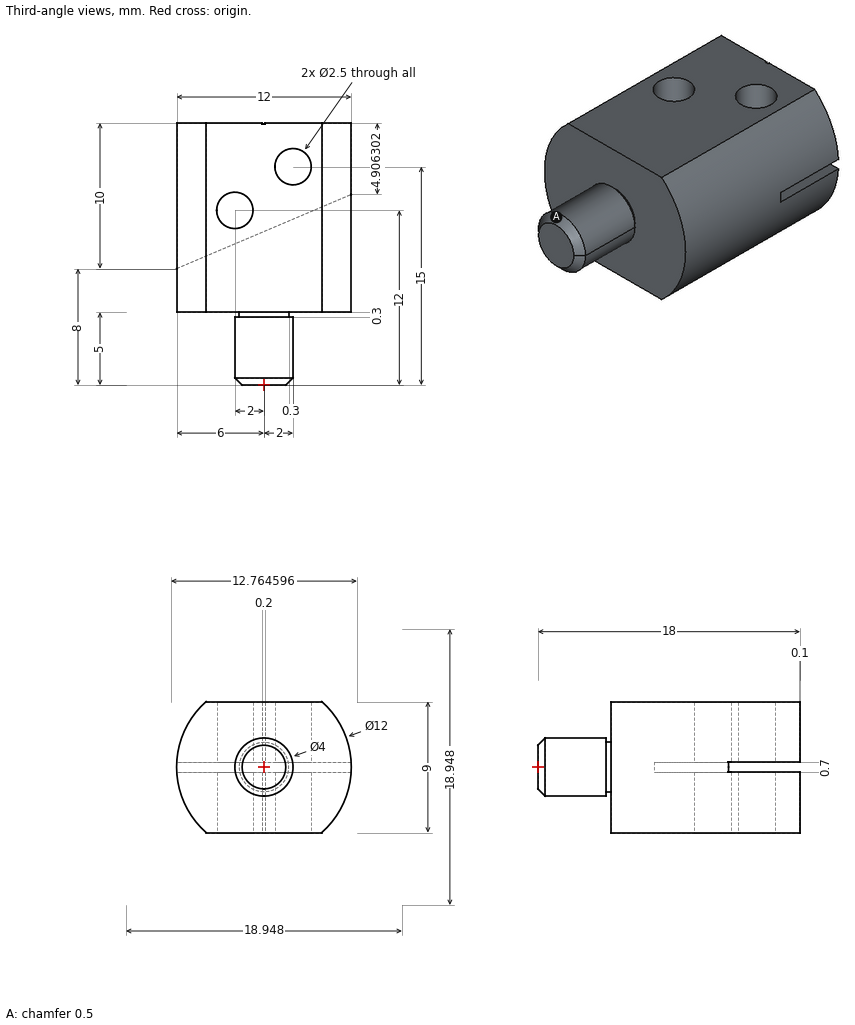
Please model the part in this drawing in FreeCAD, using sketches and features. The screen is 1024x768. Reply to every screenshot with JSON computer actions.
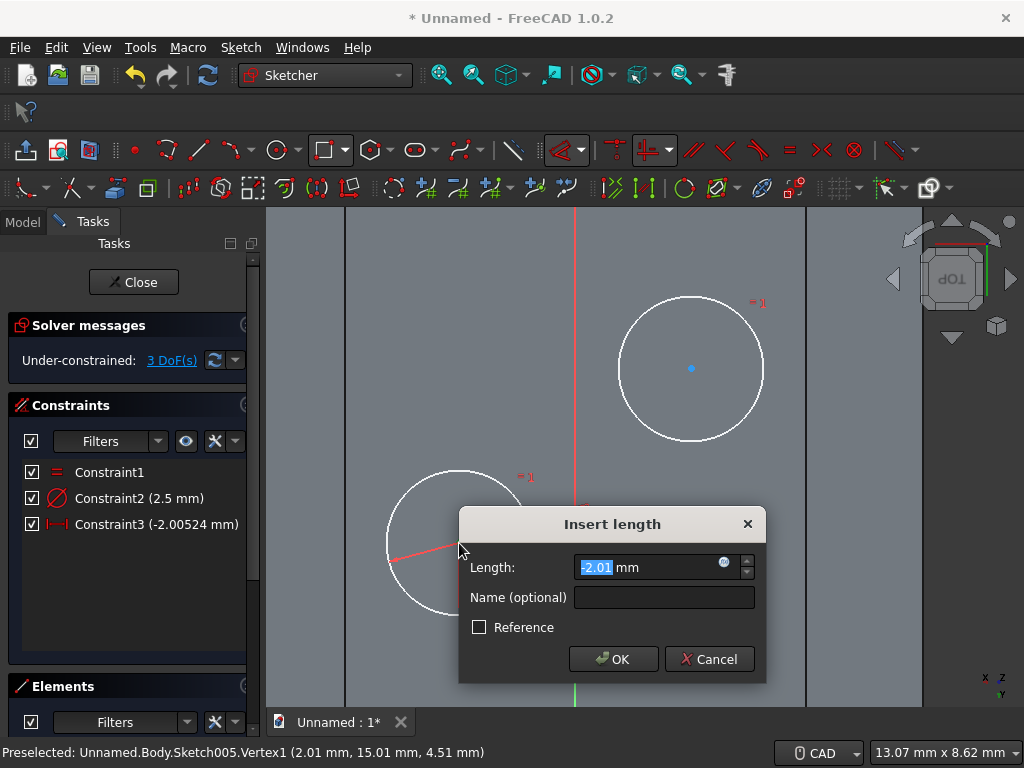
{"action": "type", "text": "-2"}
{"action": "key", "text": "Return"}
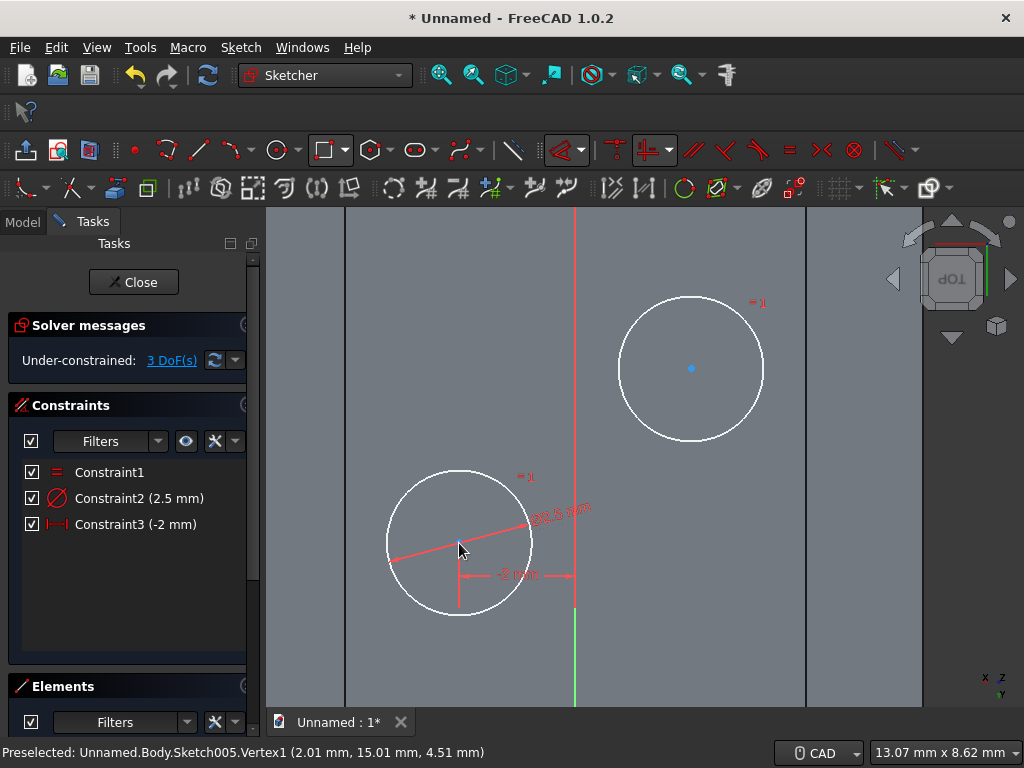
{"action": "left_click", "coordinate": [691, 369]}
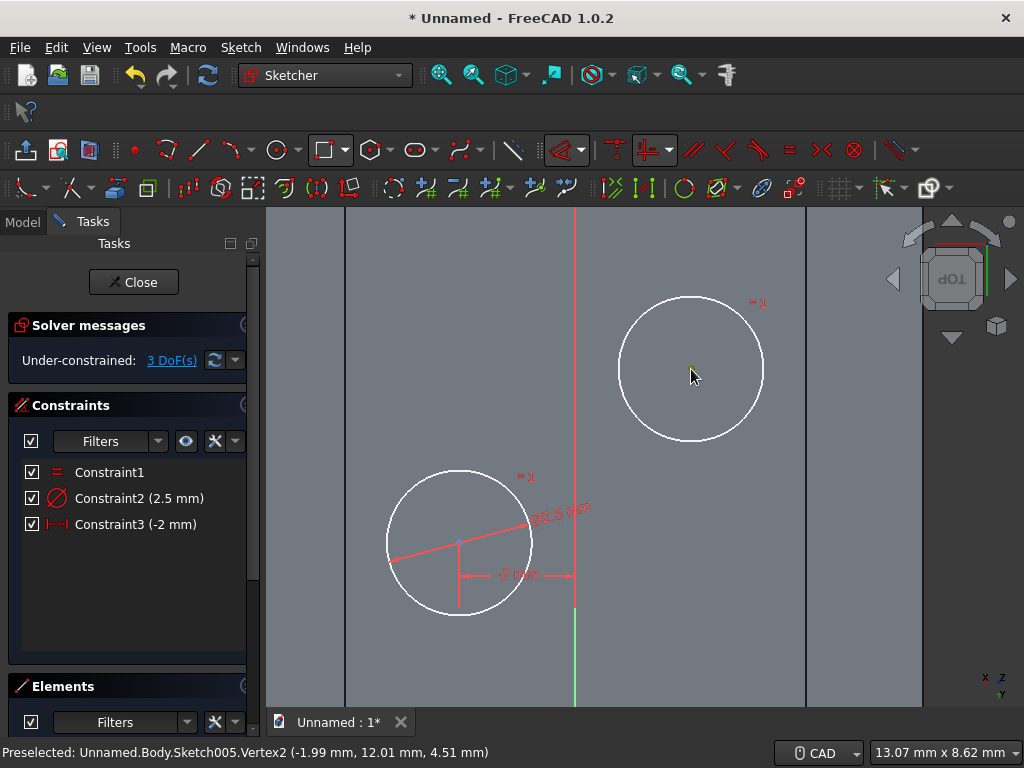
{"action": "key", "text": "l"}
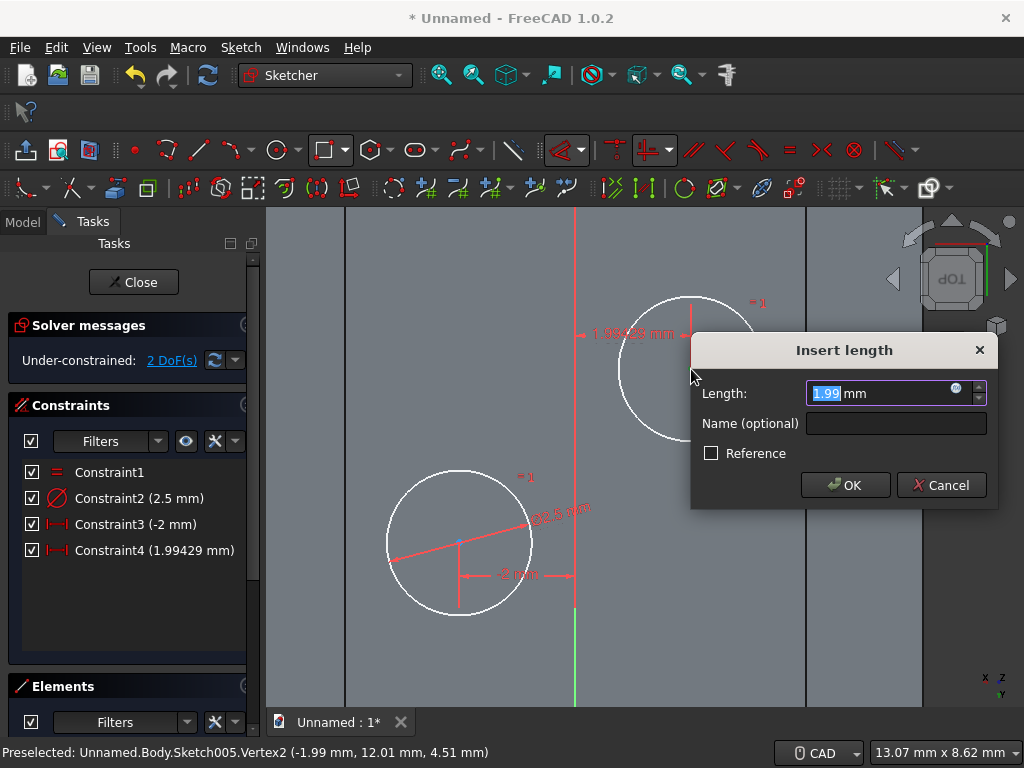
{"action": "type", "text": "2"}
{"action": "key", "text": "Return"}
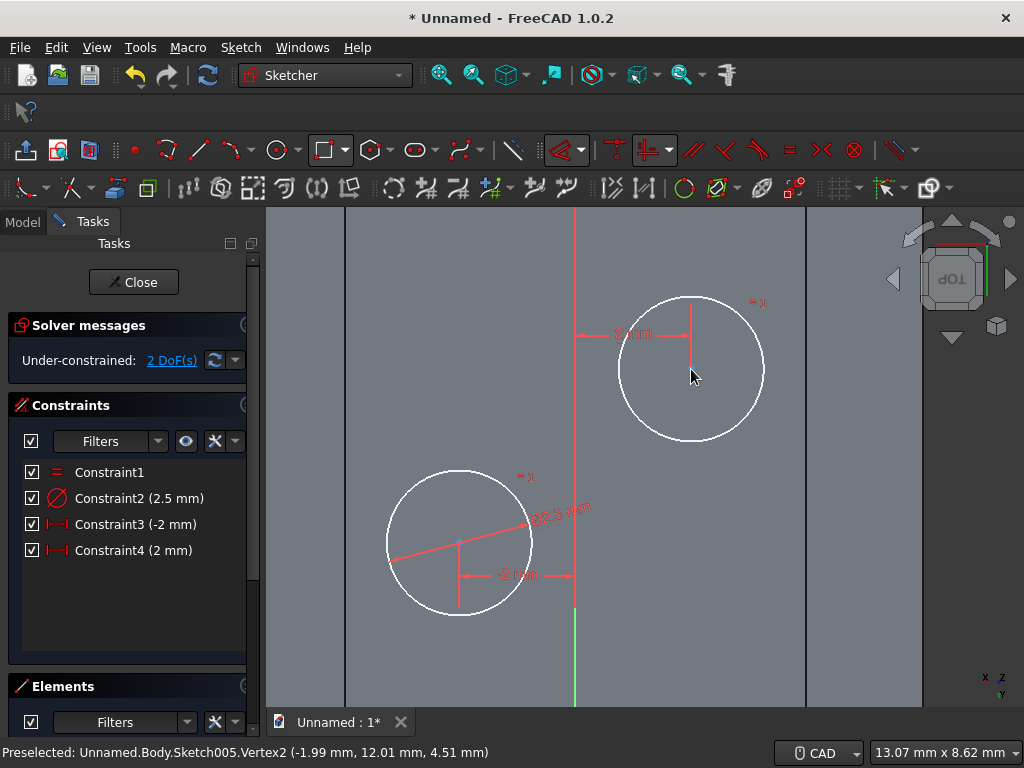
{"action": "left_click", "coordinate": [459, 543]}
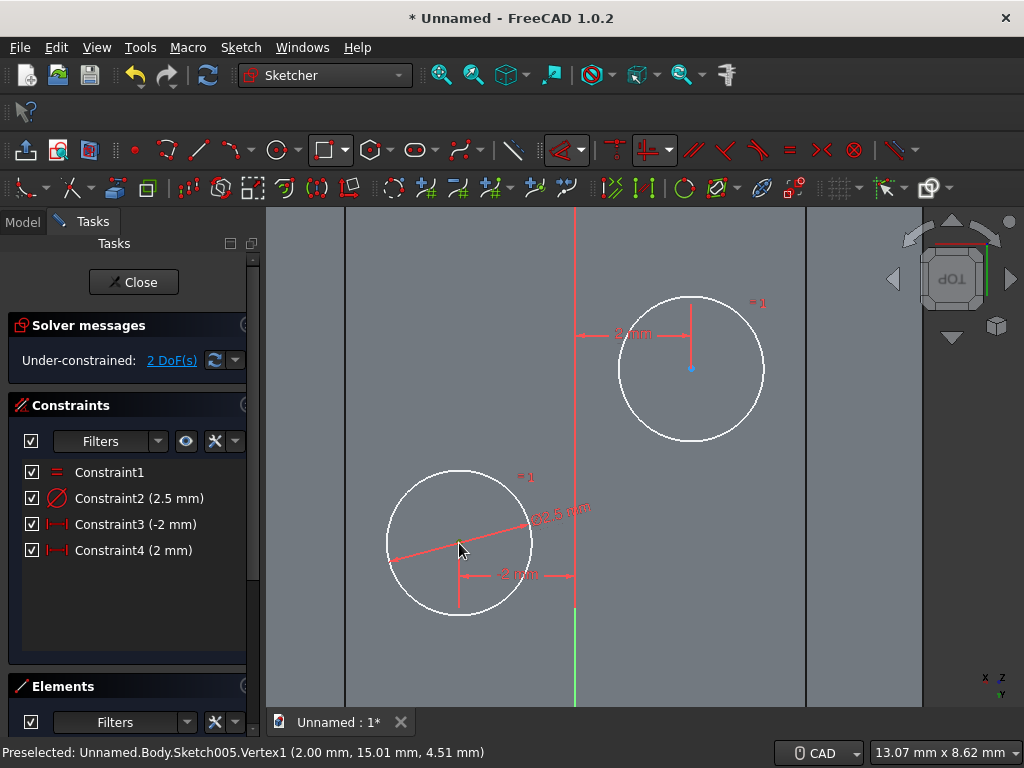
{"action": "key", "text": "i"}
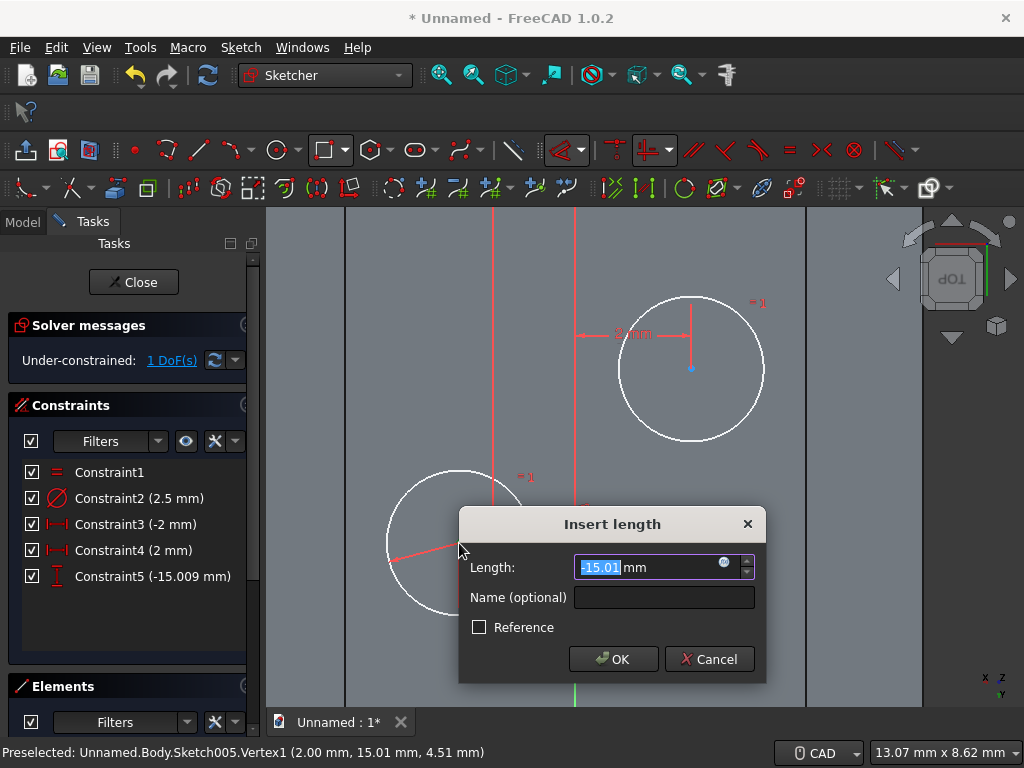
{"action": "type", "text": "-15"}
{"action": "key", "text": "Return"}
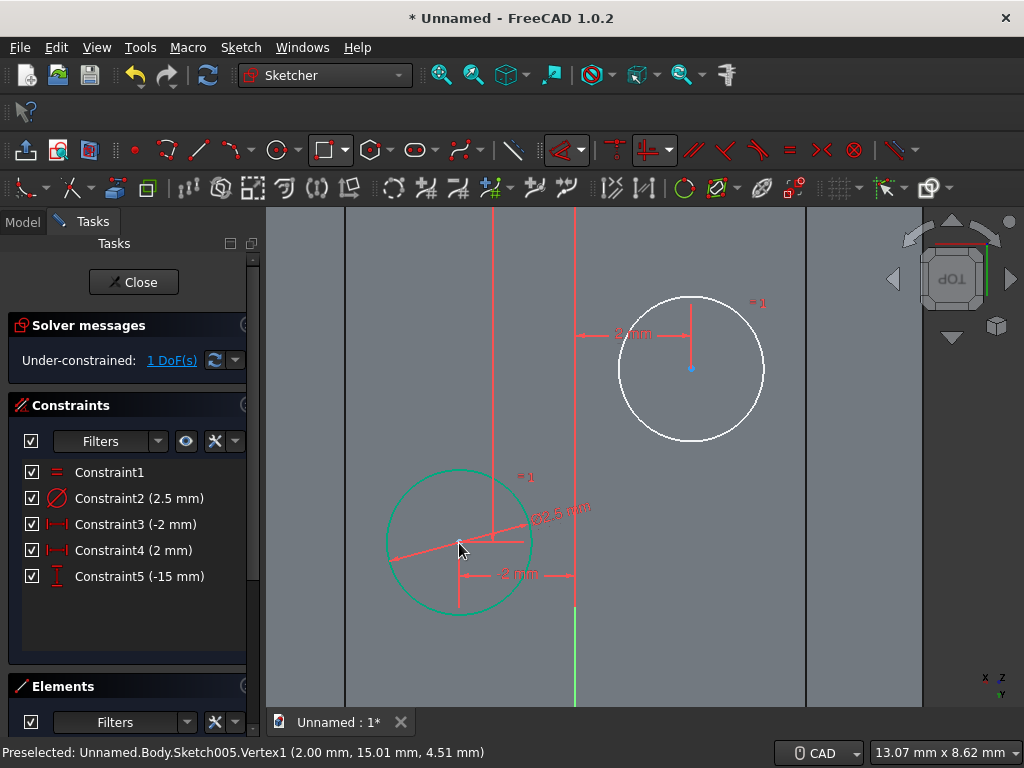
{"action": "left_click", "coordinate": [691, 369]}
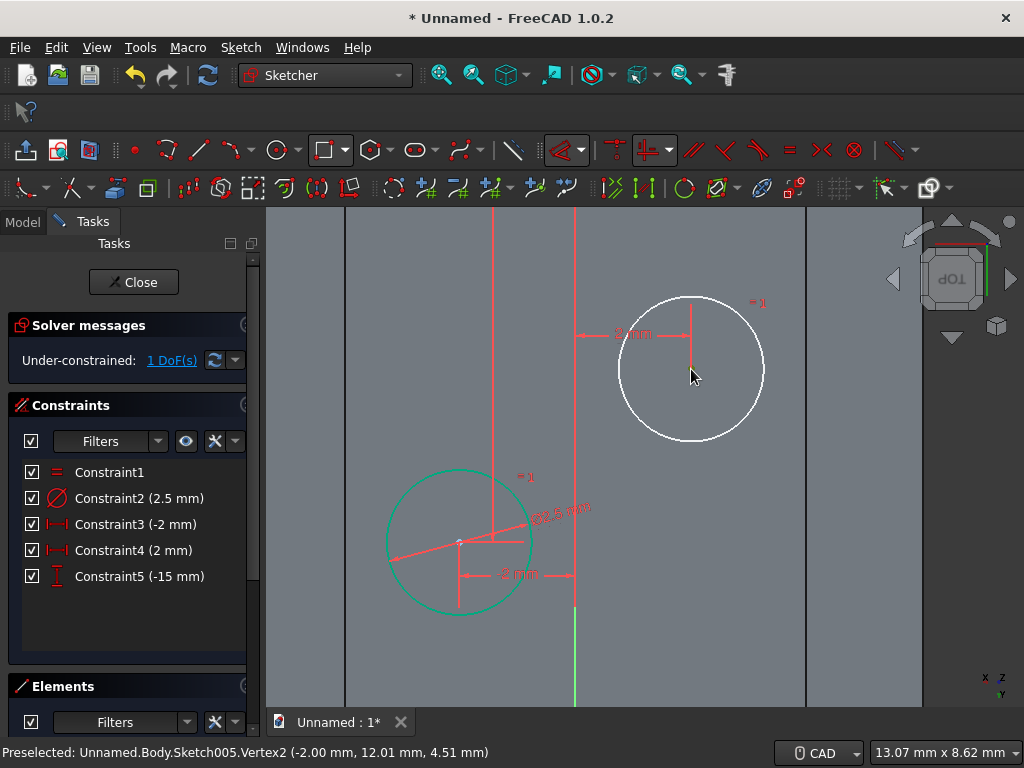
{"action": "key", "text": "i"}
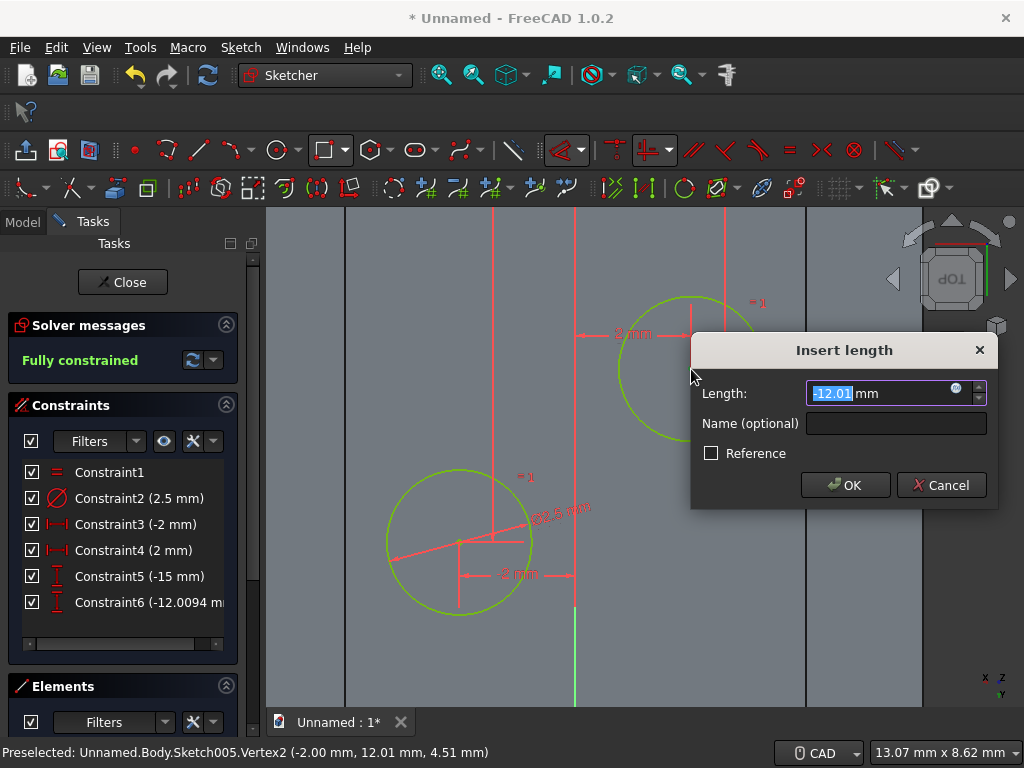
{"action": "type", "text": "-12"}
{"action": "key", "text": "Return"}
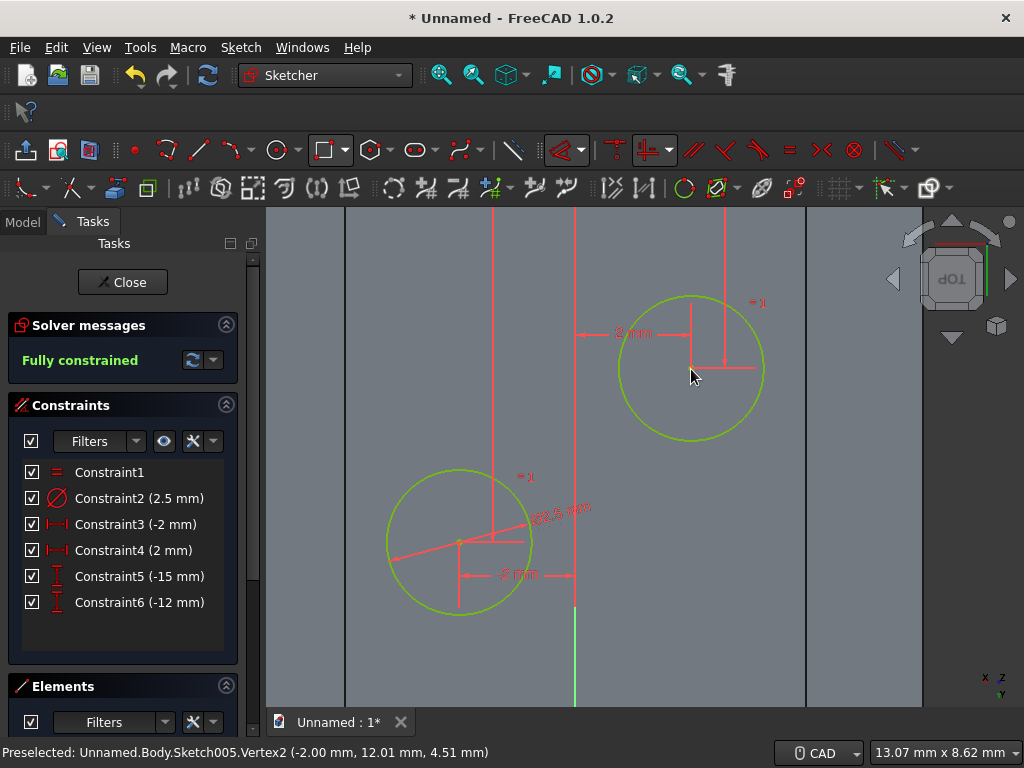
{"action": "left_click", "coordinate": [123, 282]}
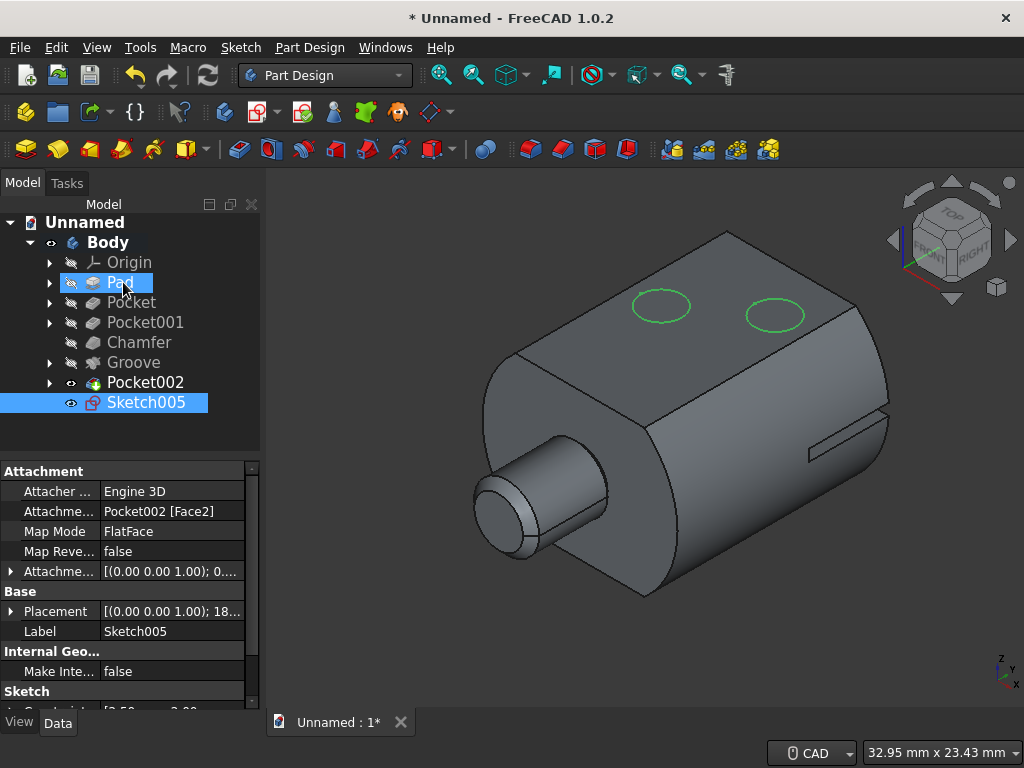
{"action": "left_click", "coordinate": [272, 150]}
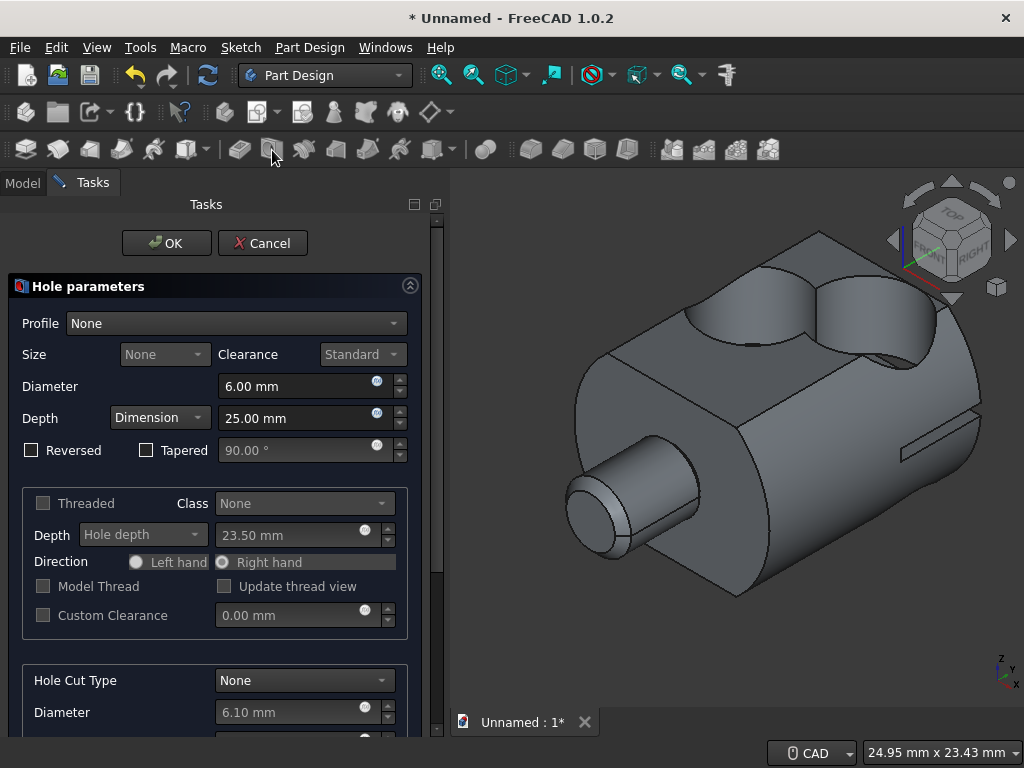
{"action": "triple_click", "coordinate": [305, 386]}